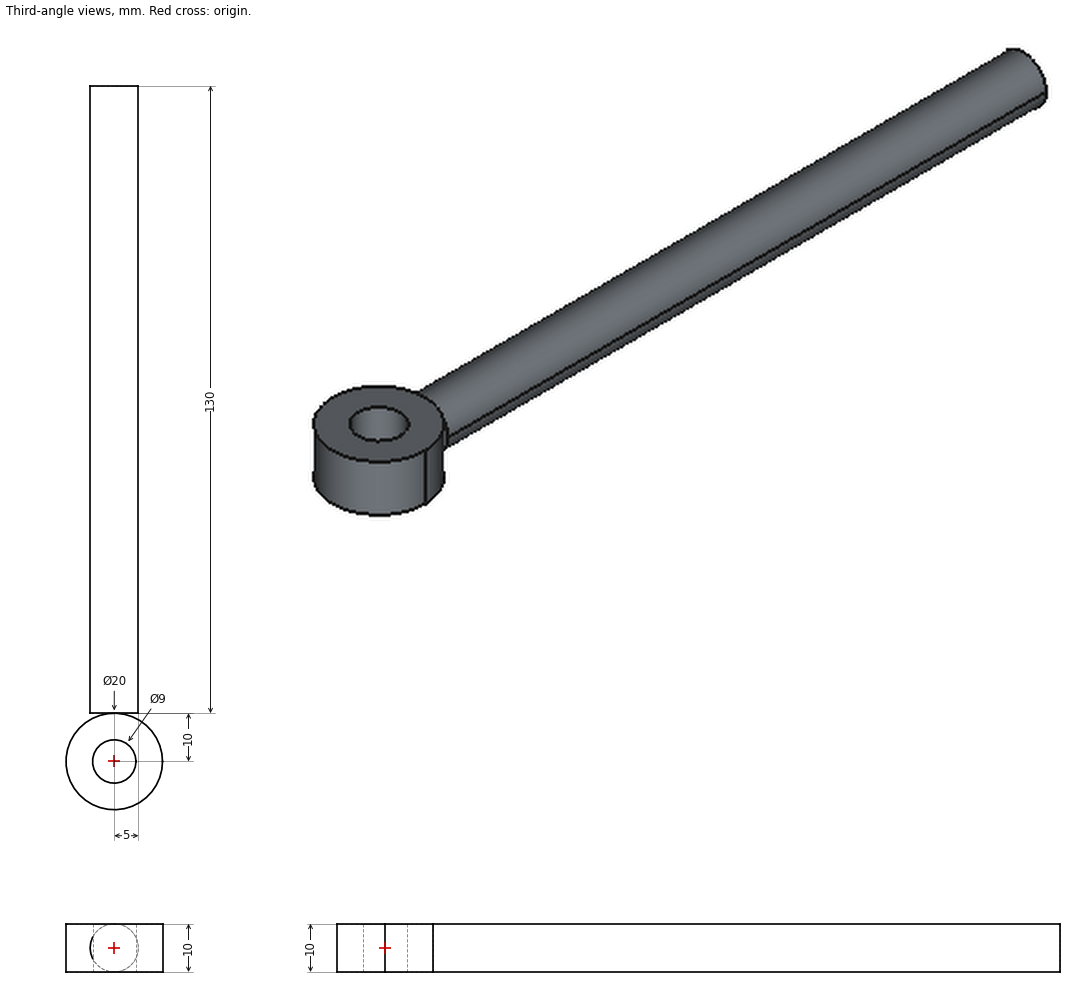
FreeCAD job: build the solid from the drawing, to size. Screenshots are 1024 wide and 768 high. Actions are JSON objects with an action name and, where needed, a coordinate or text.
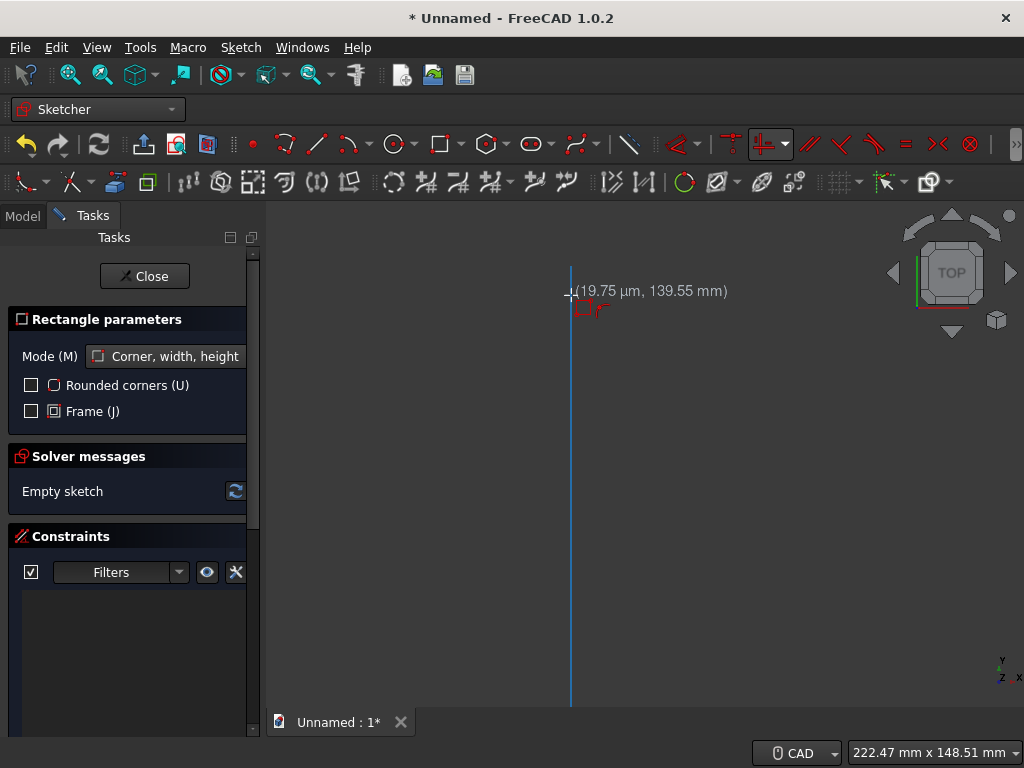
{"action": "left_click", "coordinate": [571, 295]}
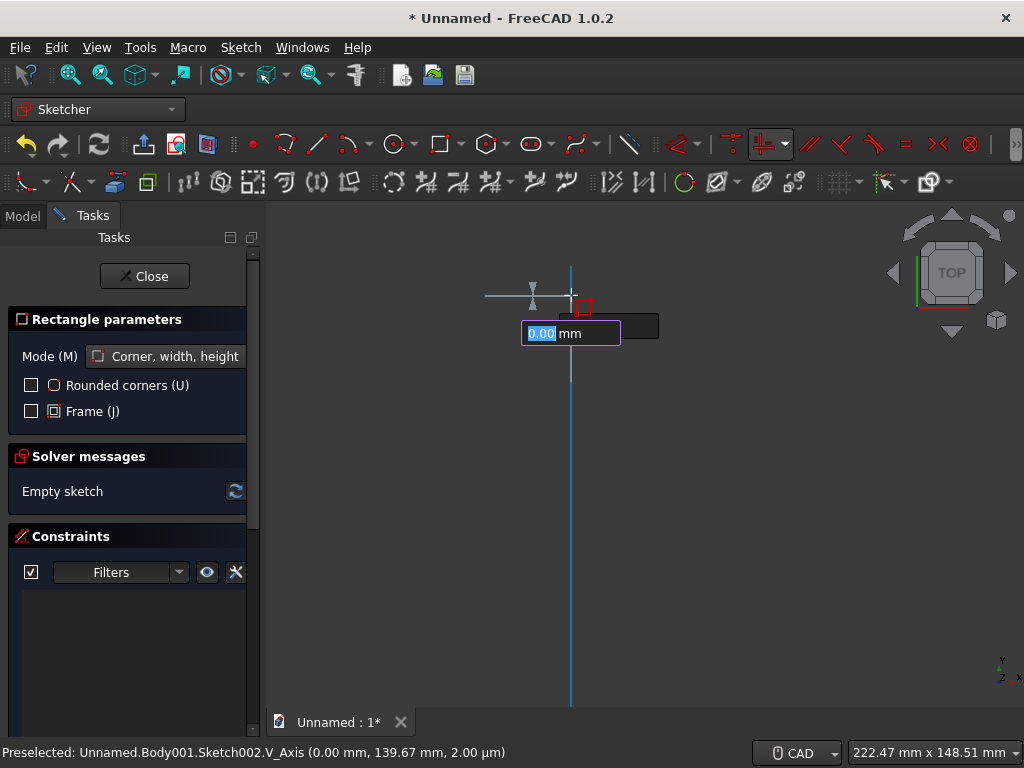
{"action": "scroll", "coordinate": [571, 293], "scroll_direction": "down", "scroll_amount": 2}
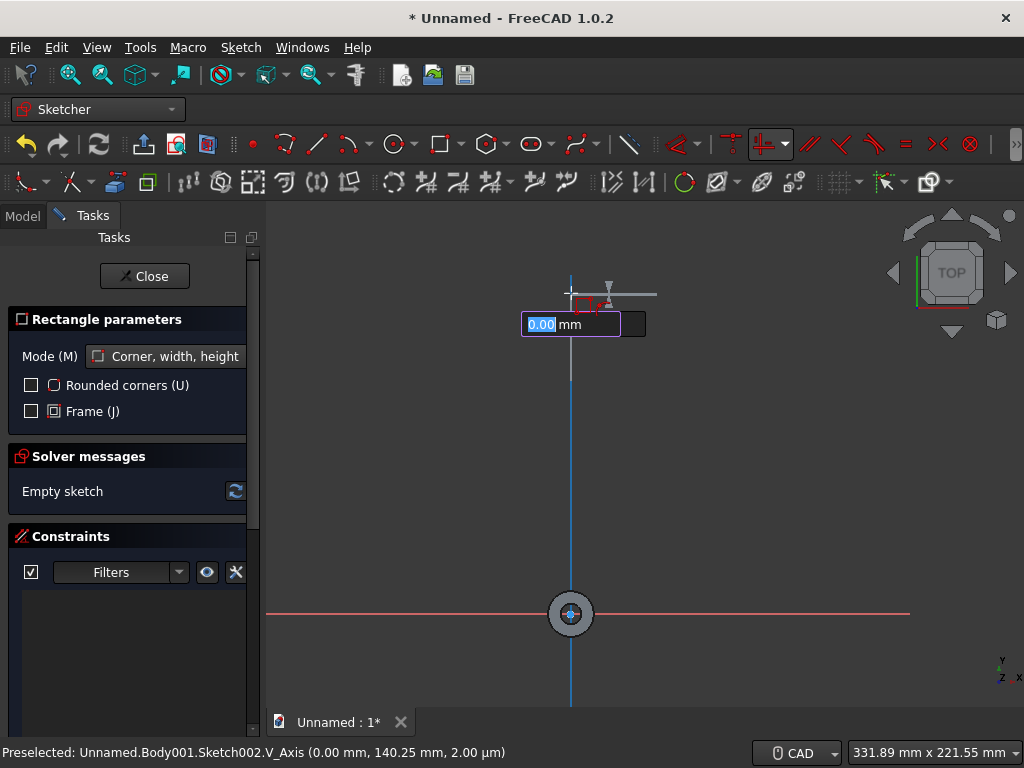
{"action": "scroll", "coordinate": [582, 591], "scroll_direction": "up", "scroll_amount": 2}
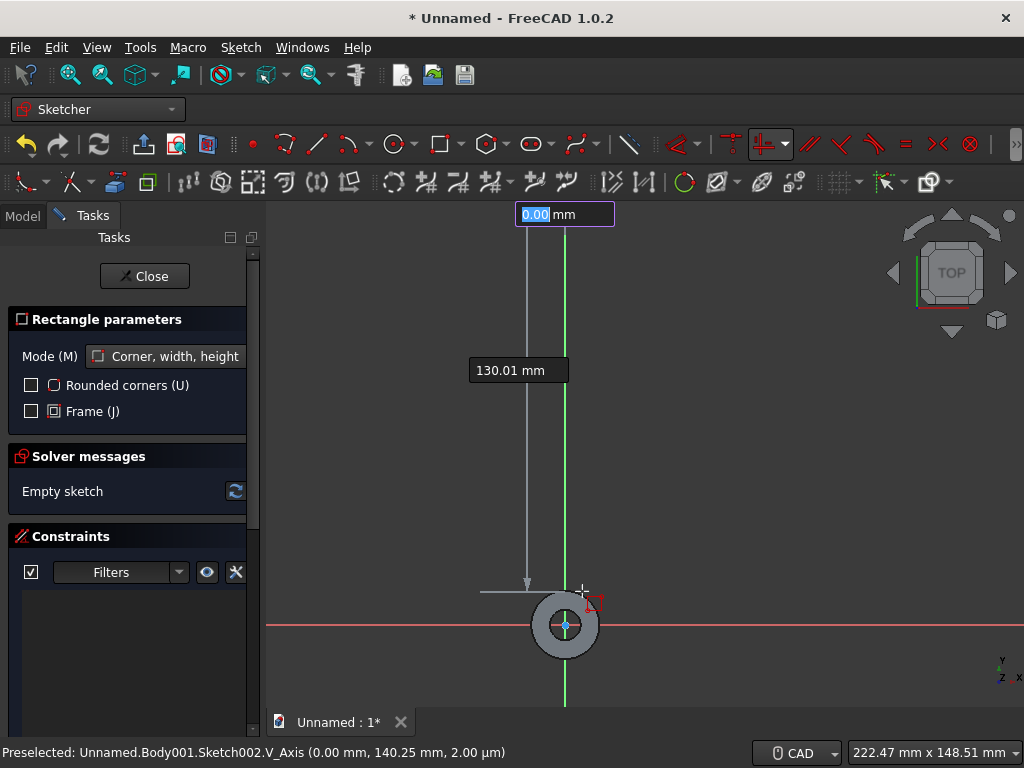
{"action": "left_click", "coordinate": [582, 591]}
{"action": "key", "text": "Escape"}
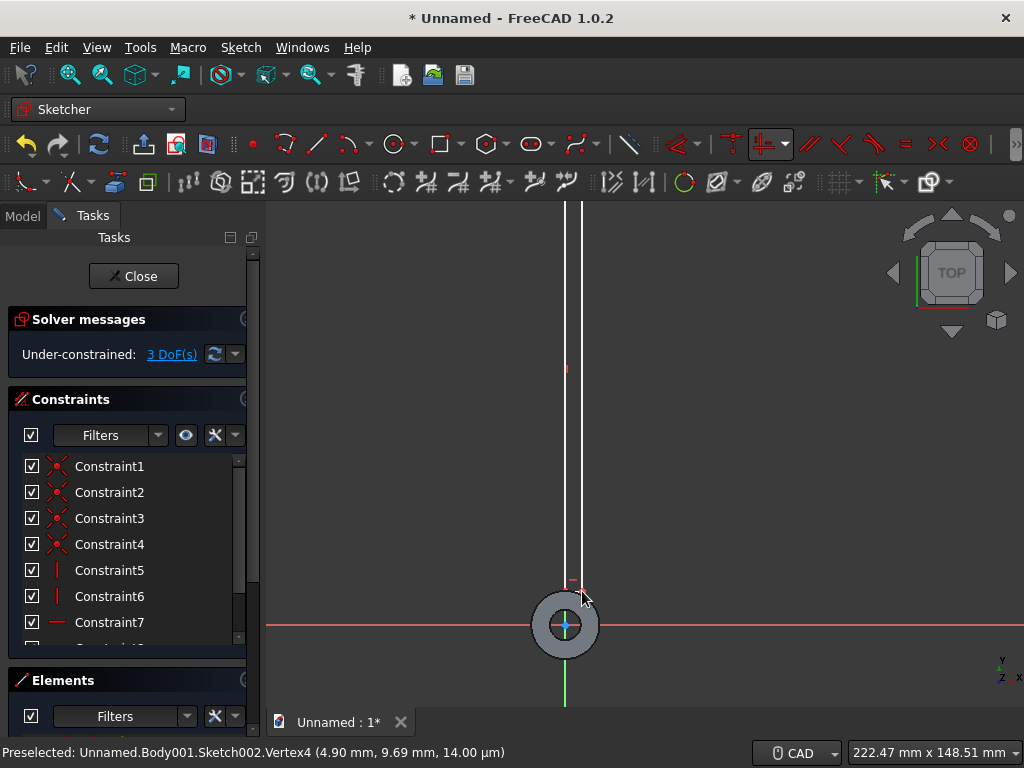
{"action": "left_click", "coordinate": [676, 144]}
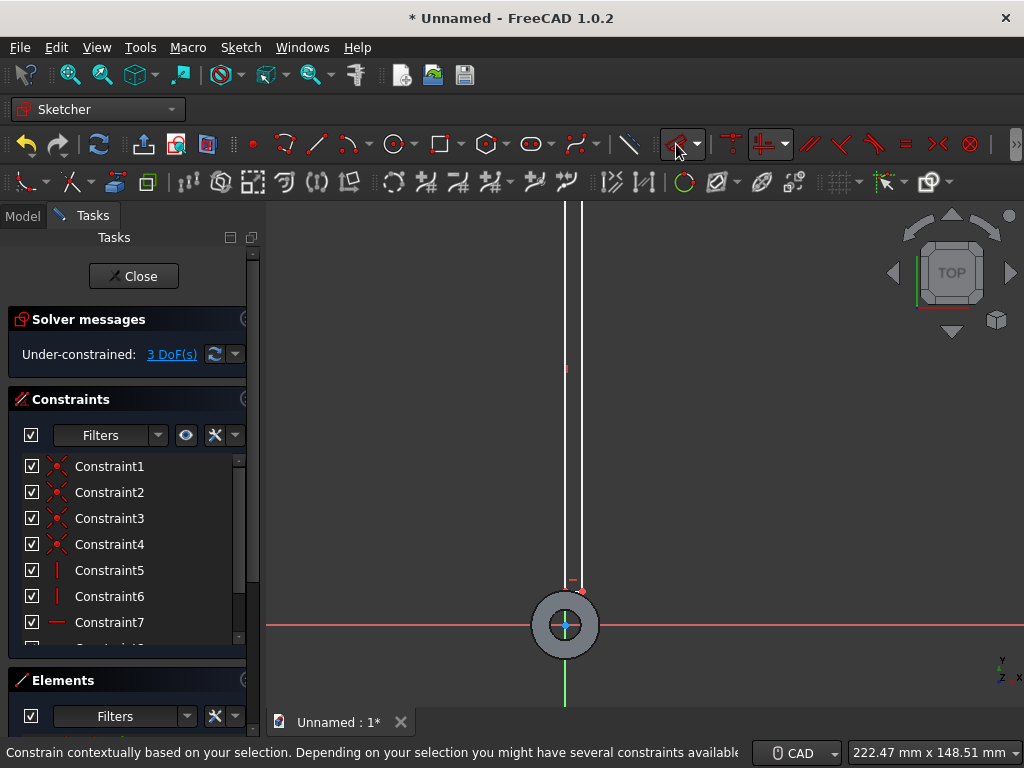
{"action": "scroll", "coordinate": [574, 592], "scroll_direction": "up", "scroll_amount": 5}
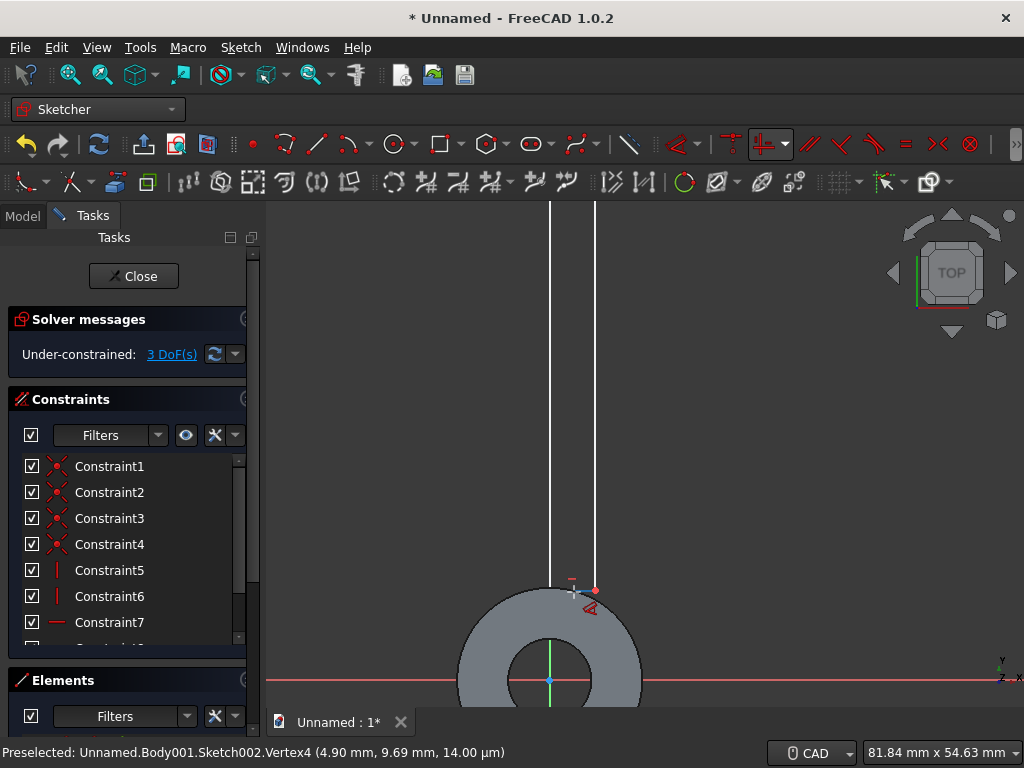
{"action": "left_click", "coordinate": [572, 591]}
{"action": "left_click", "coordinate": [572, 625]}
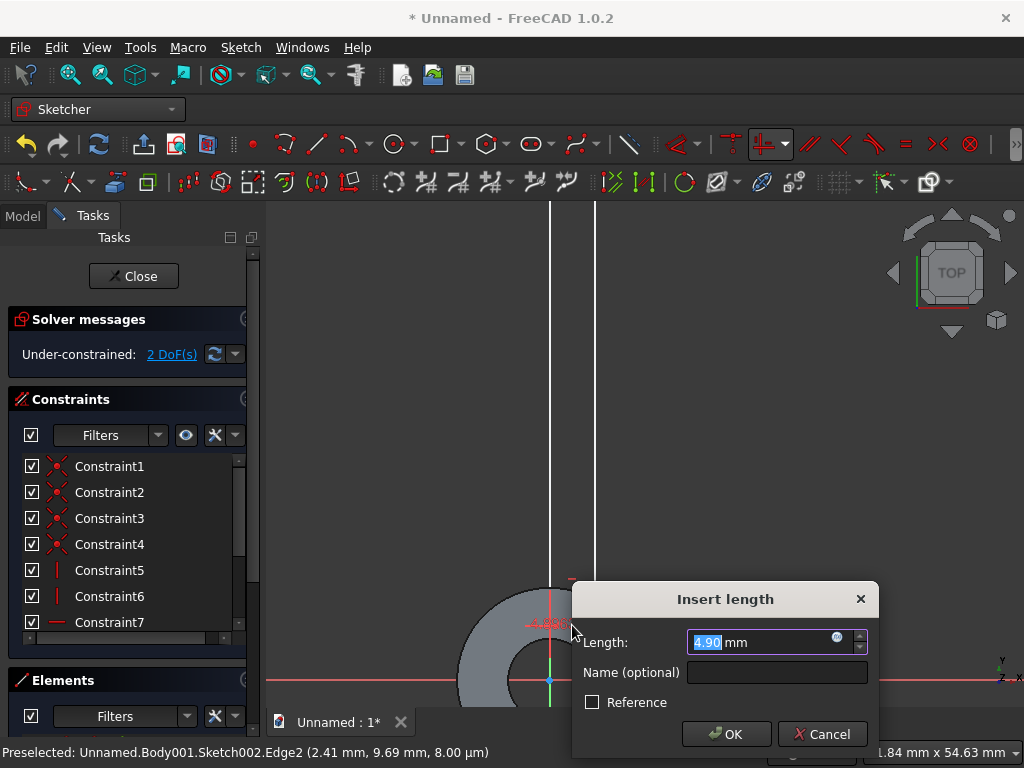
{"action": "type", "text": "5"}
{"action": "key", "text": "Return"}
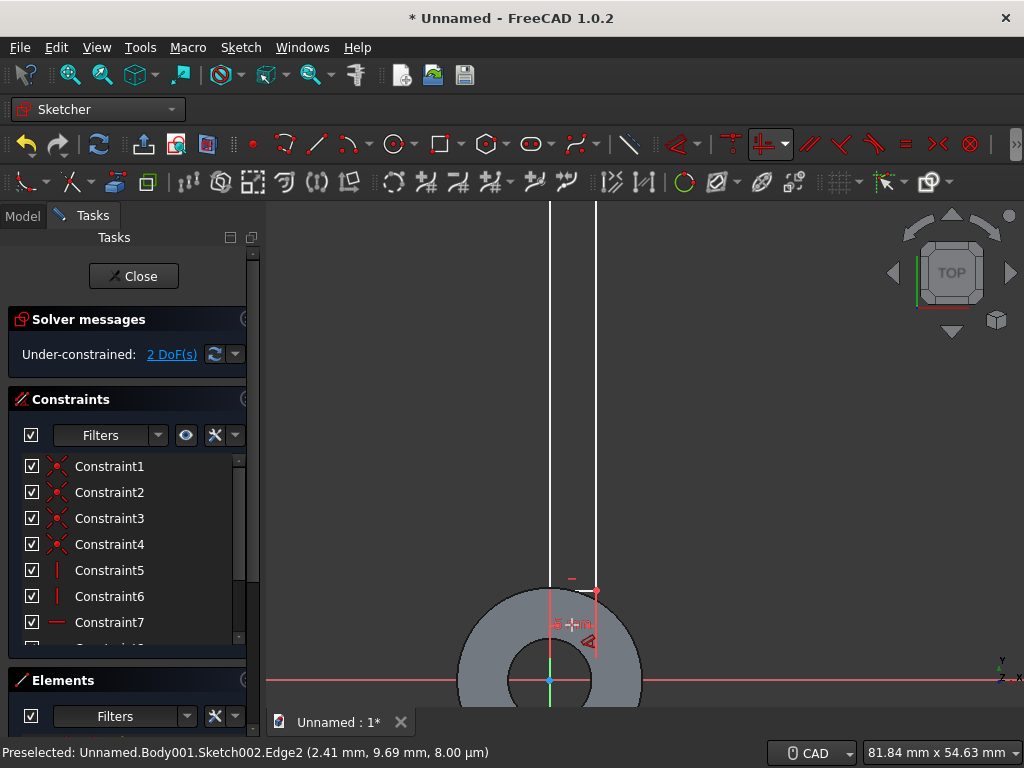
{"action": "scroll", "coordinate": [578, 592], "scroll_direction": "down", "scroll_amount": 7}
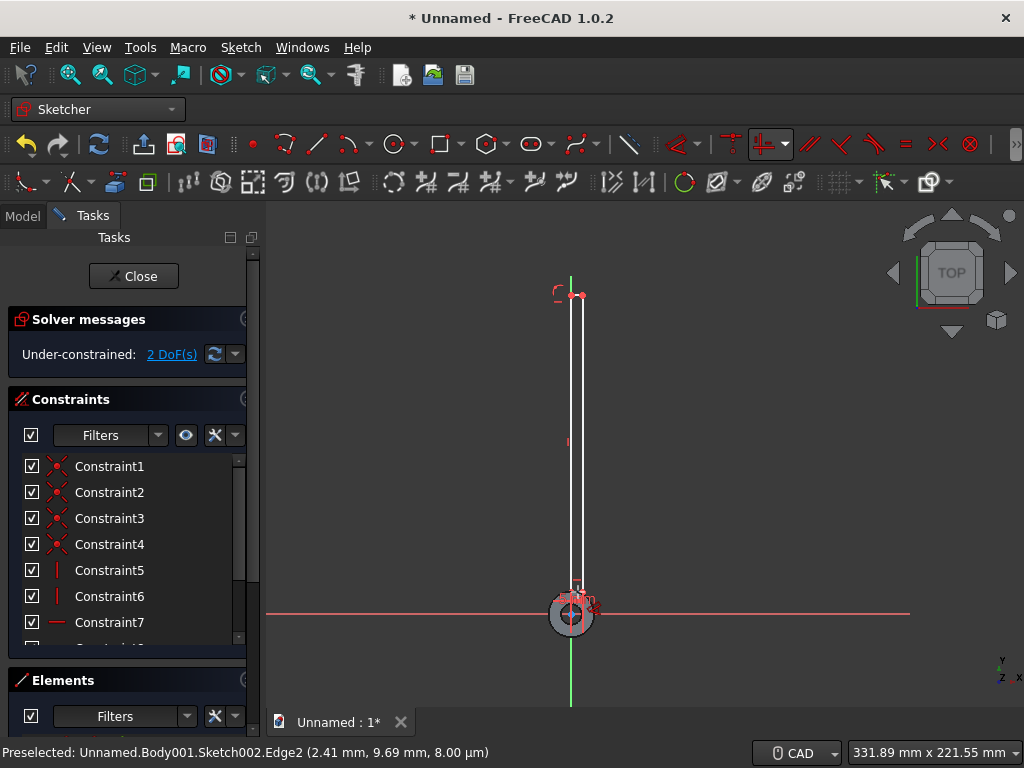
{"action": "left_click", "coordinate": [571, 503]}
{"action": "left_click", "coordinate": [537, 444]}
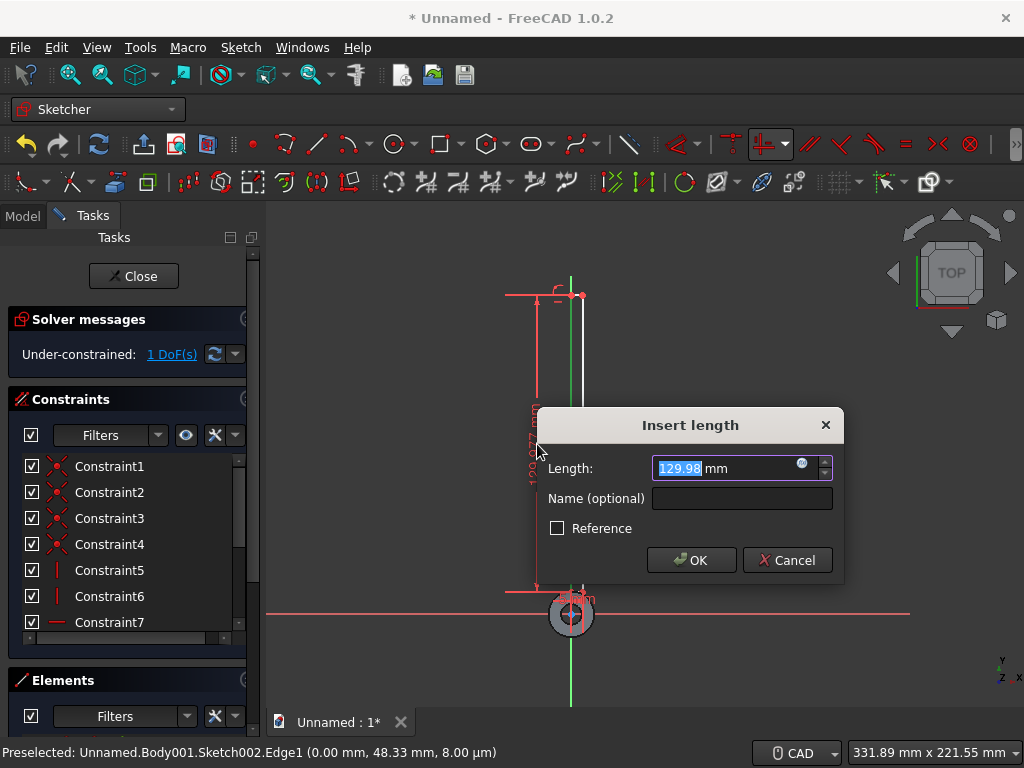
{"action": "type", "text": "130"}
{"action": "key", "text": "Return"}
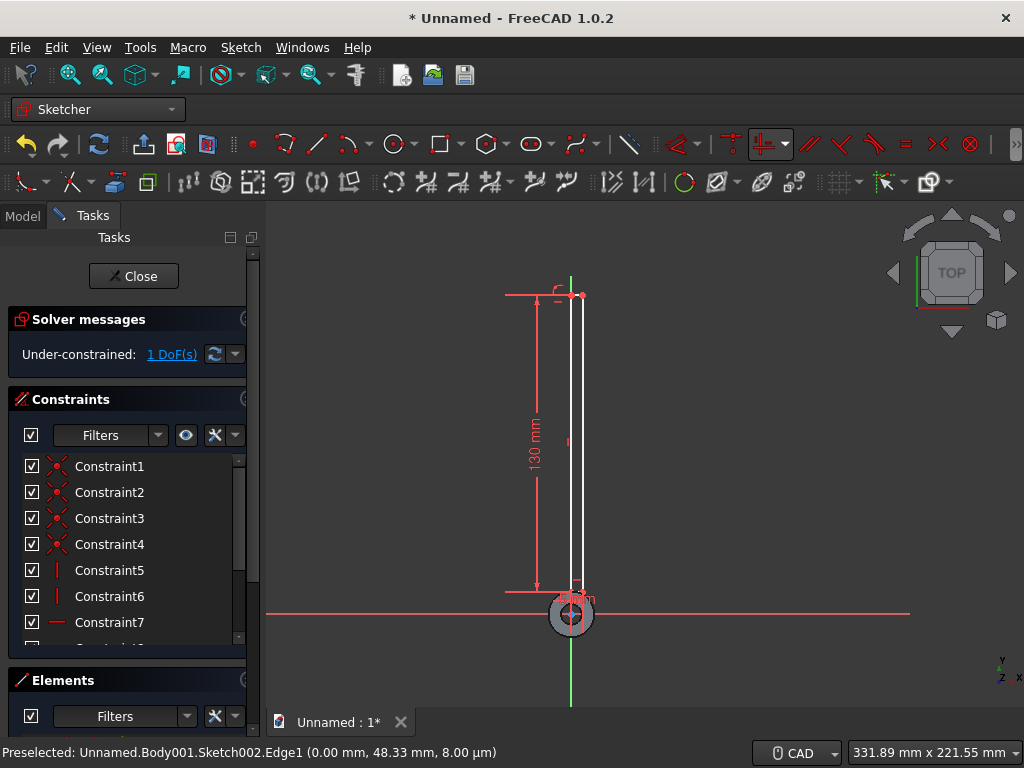
{"action": "scroll", "coordinate": [571, 592], "scroll_direction": "up", "scroll_amount": 3}